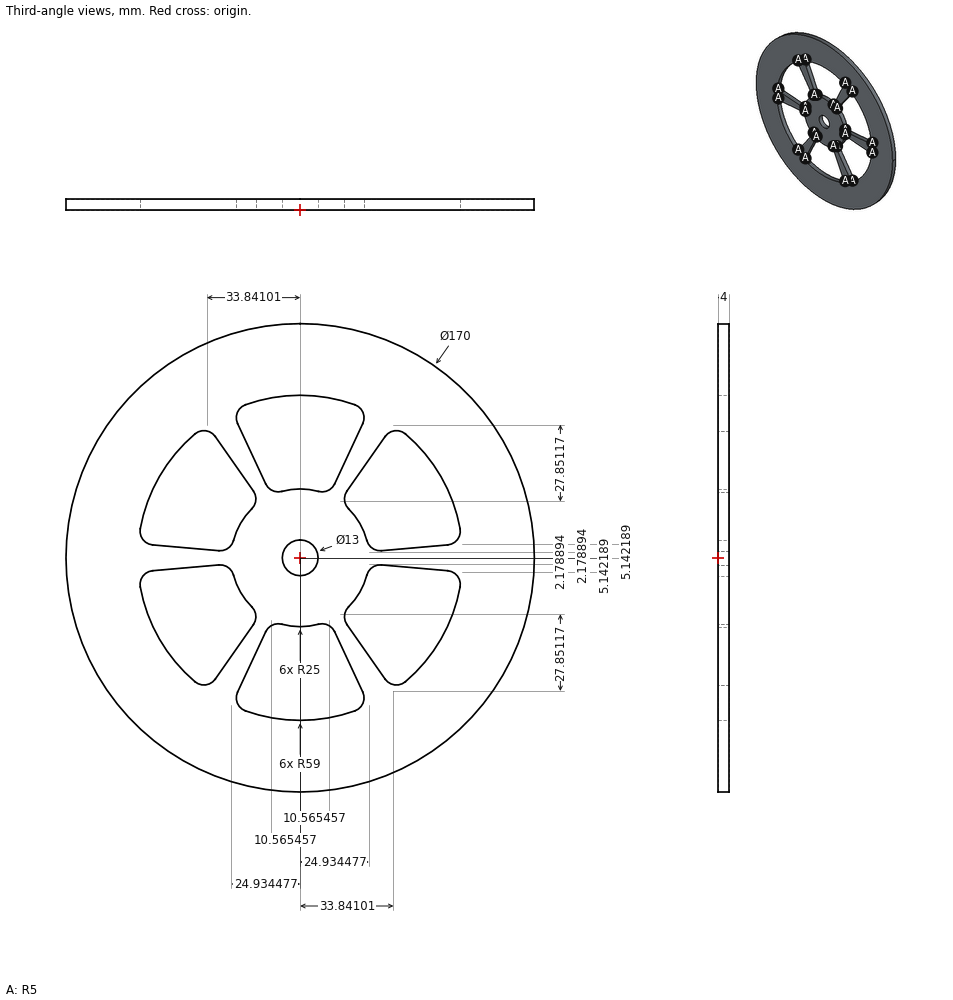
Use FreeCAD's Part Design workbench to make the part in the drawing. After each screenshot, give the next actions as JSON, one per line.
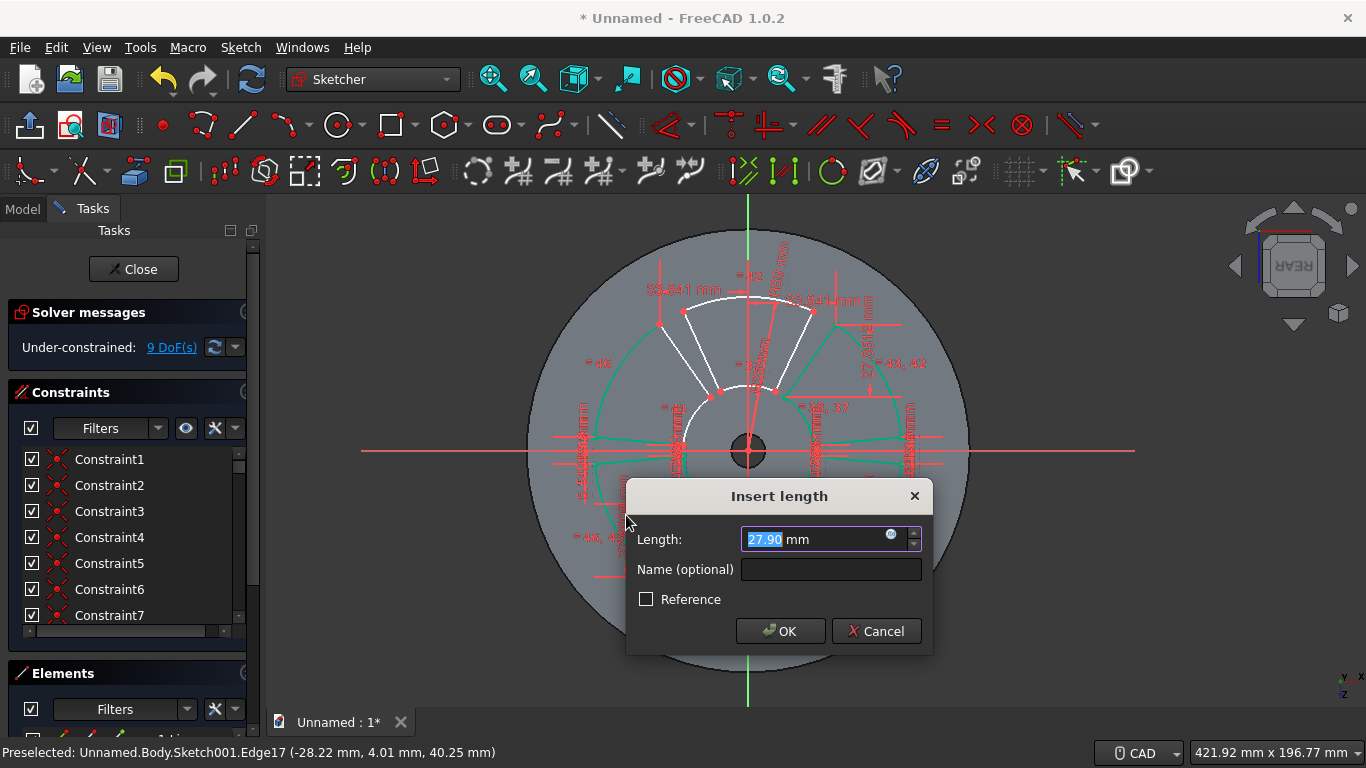
{"action": "type", "text": "27.85117"}
{"action": "key", "text": "Return"}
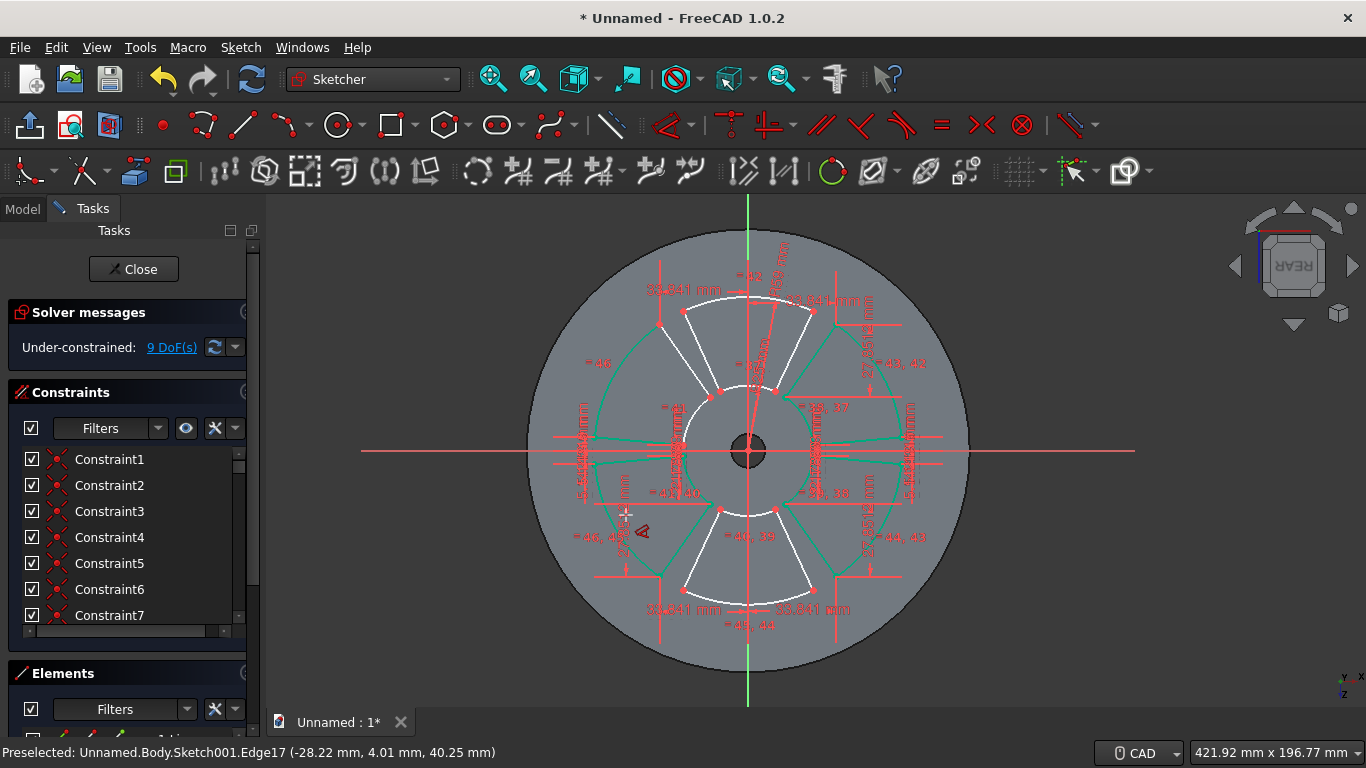
{"action": "left_click", "coordinate": [695, 376]}
{"action": "left_click", "coordinate": [626, 336]}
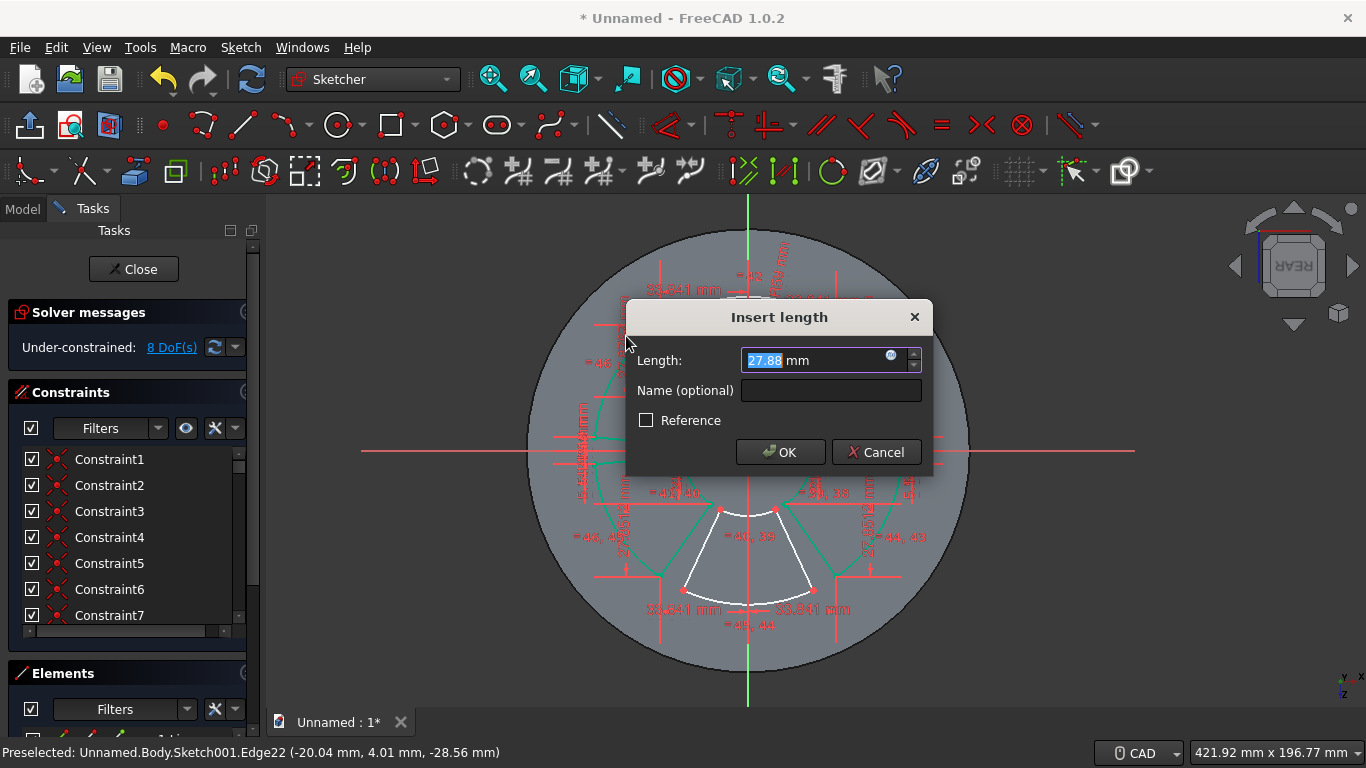
{"action": "type", "text": "27.85117"}
{"action": "key", "text": "Return"}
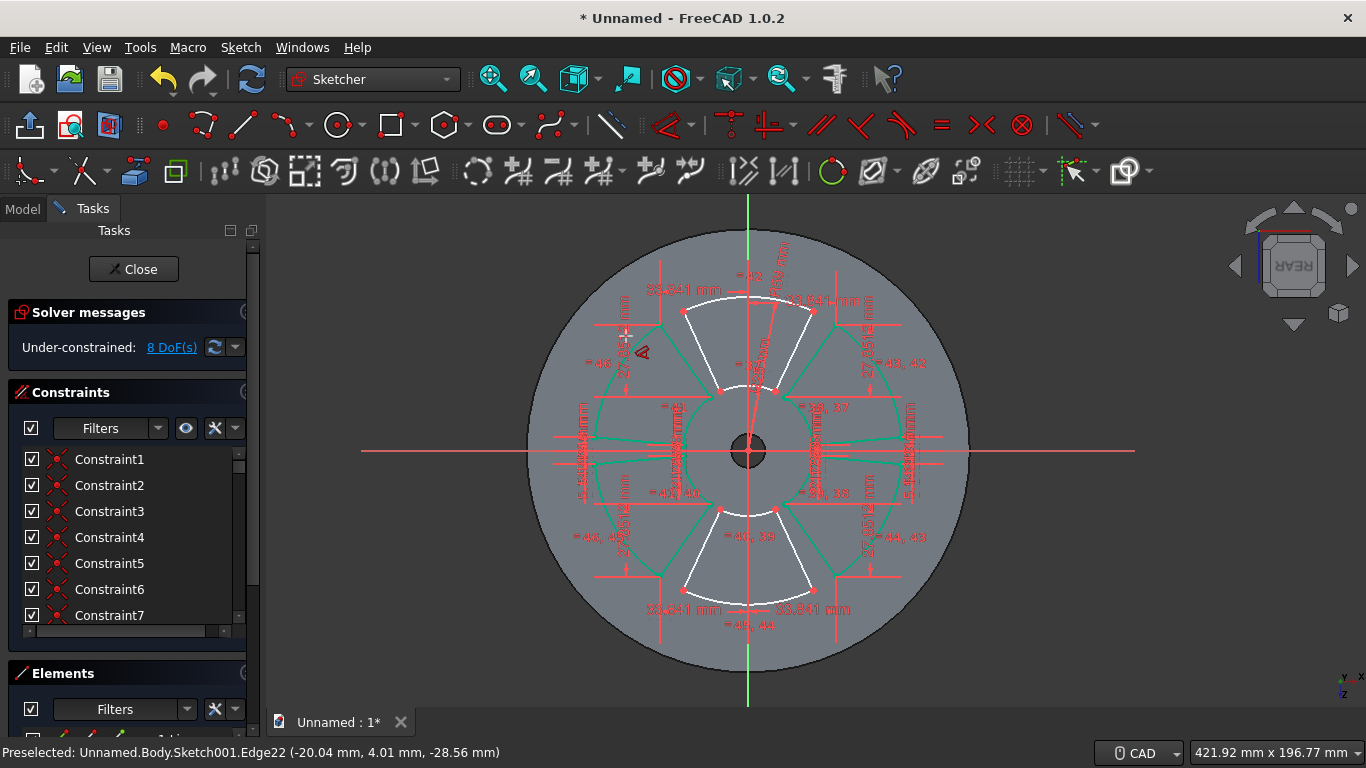
{"action": "scroll", "coordinate": [775, 392], "scroll_direction": "up", "scroll_amount": 2}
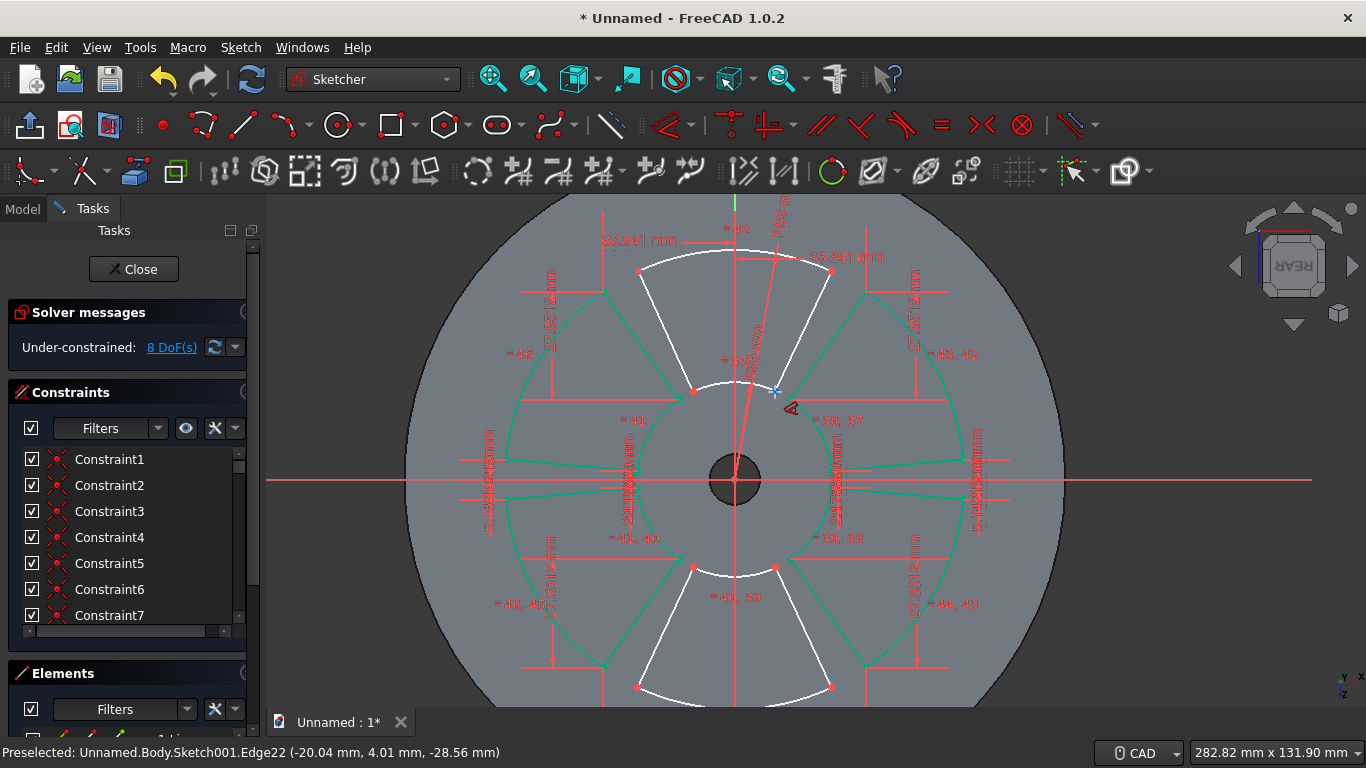
{"action": "left_click", "coordinate": [775, 391]}
{"action": "left_click", "coordinate": [755, 514]}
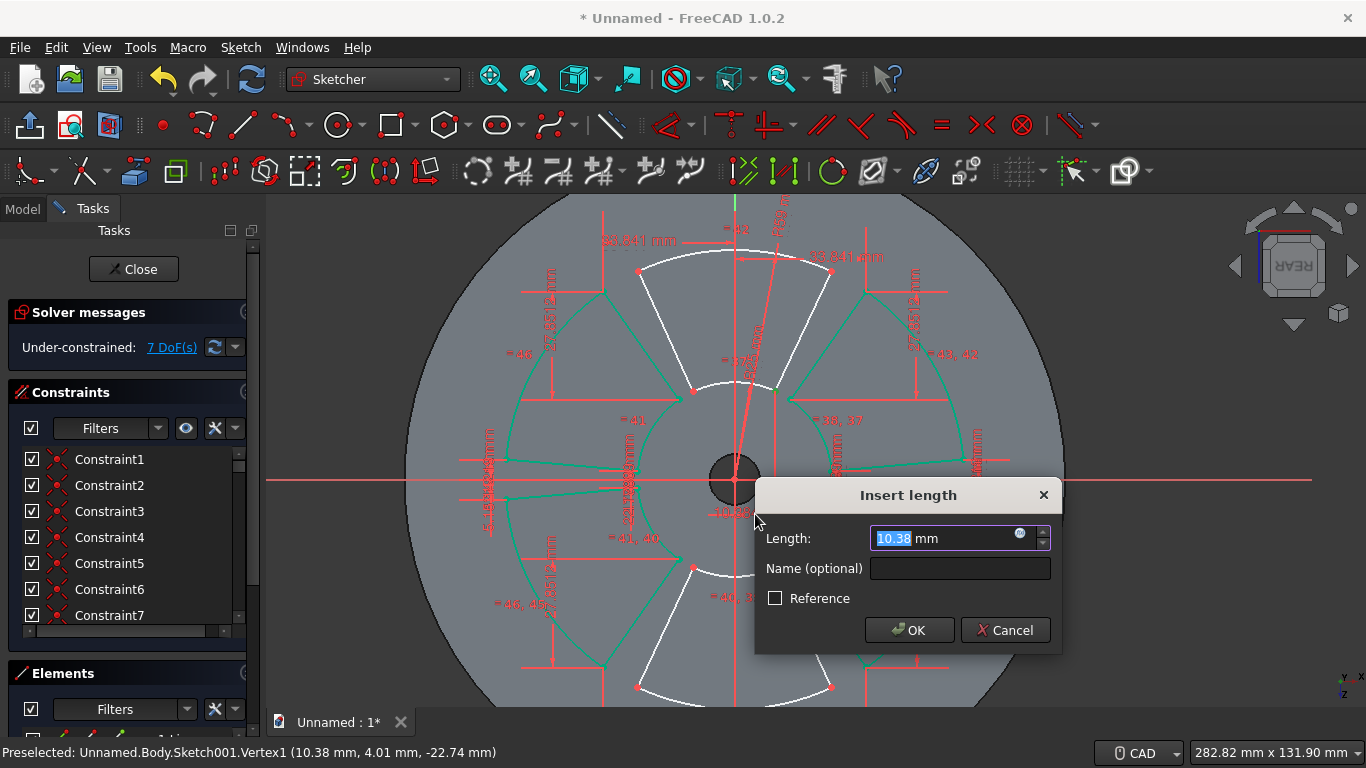
{"action": "type", "text": "10.565457"}
{"action": "key", "text": "Return"}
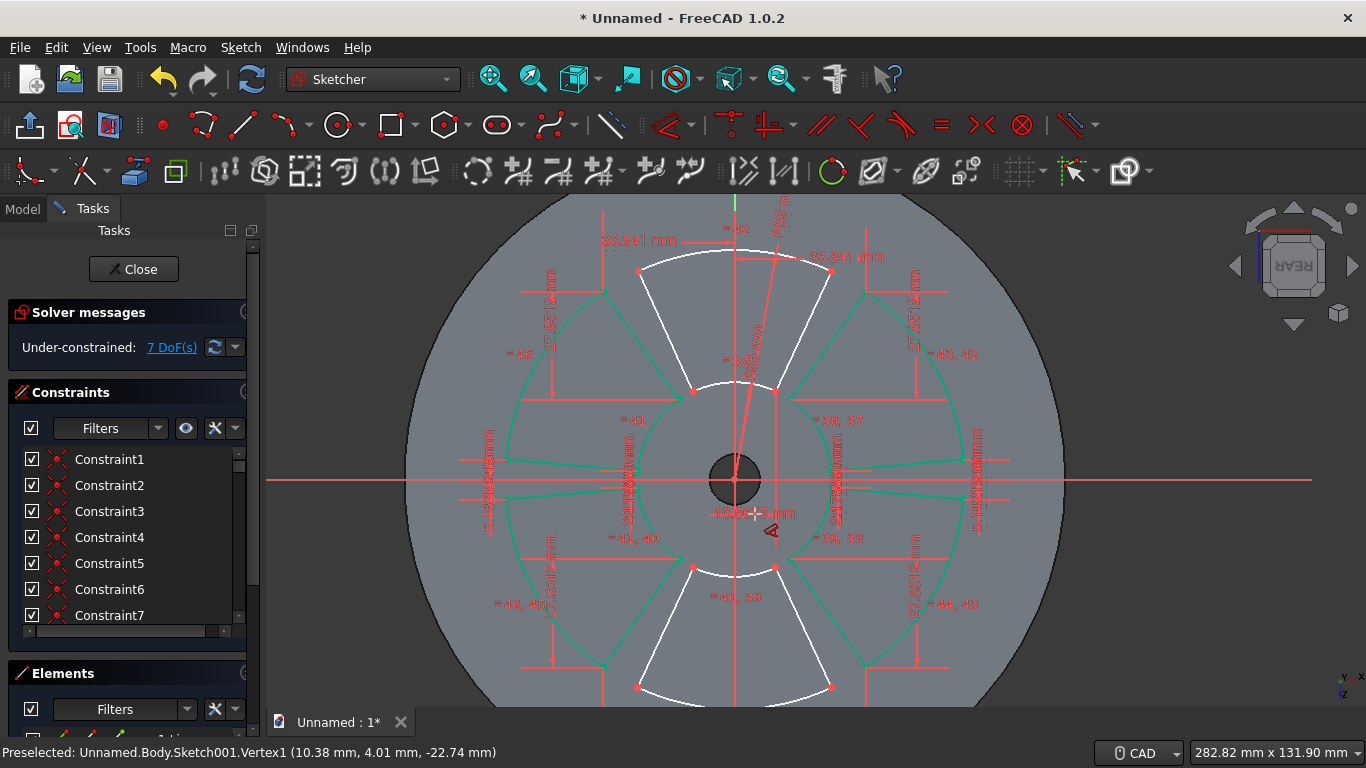
{"action": "left_click", "coordinate": [832, 271]}
{"action": "left_click", "coordinate": [783, 237]}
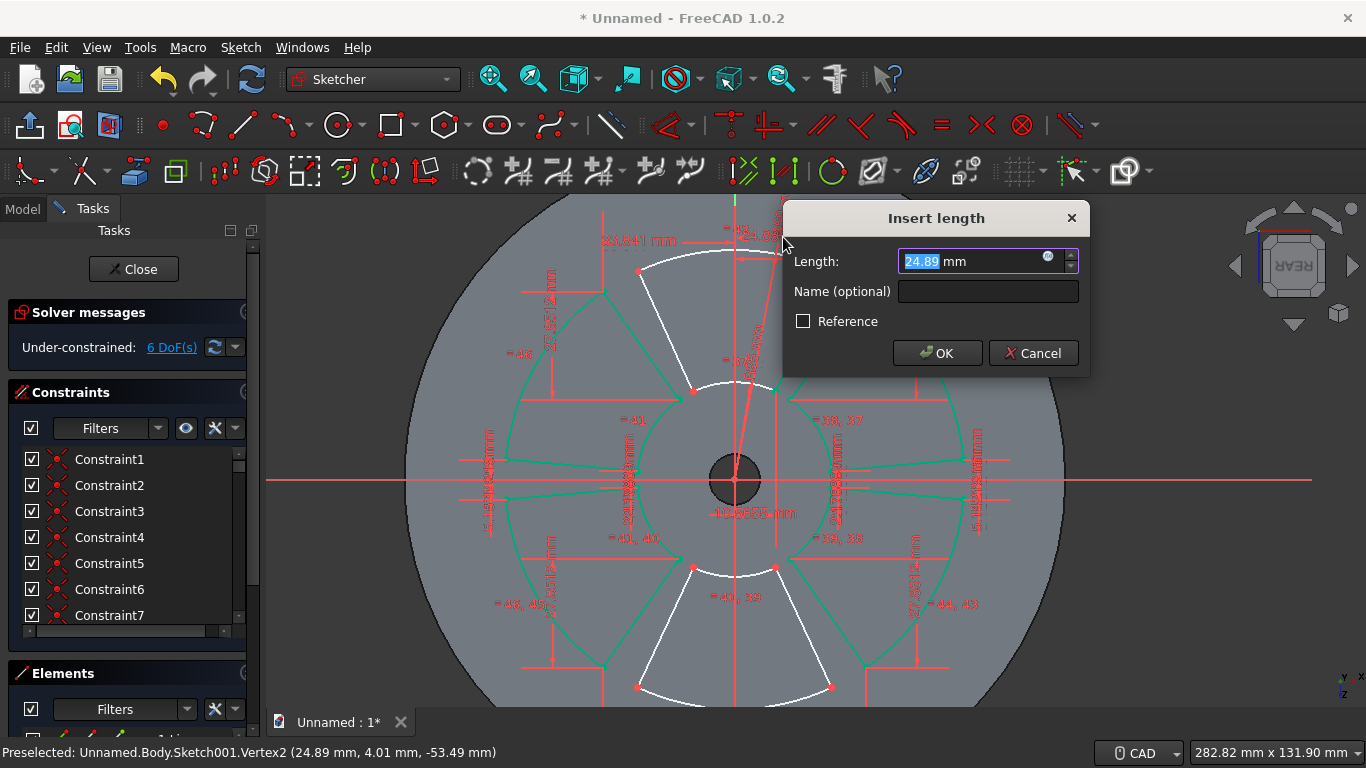
{"action": "type", "text": "24.934477"}
{"action": "key", "text": "Return"}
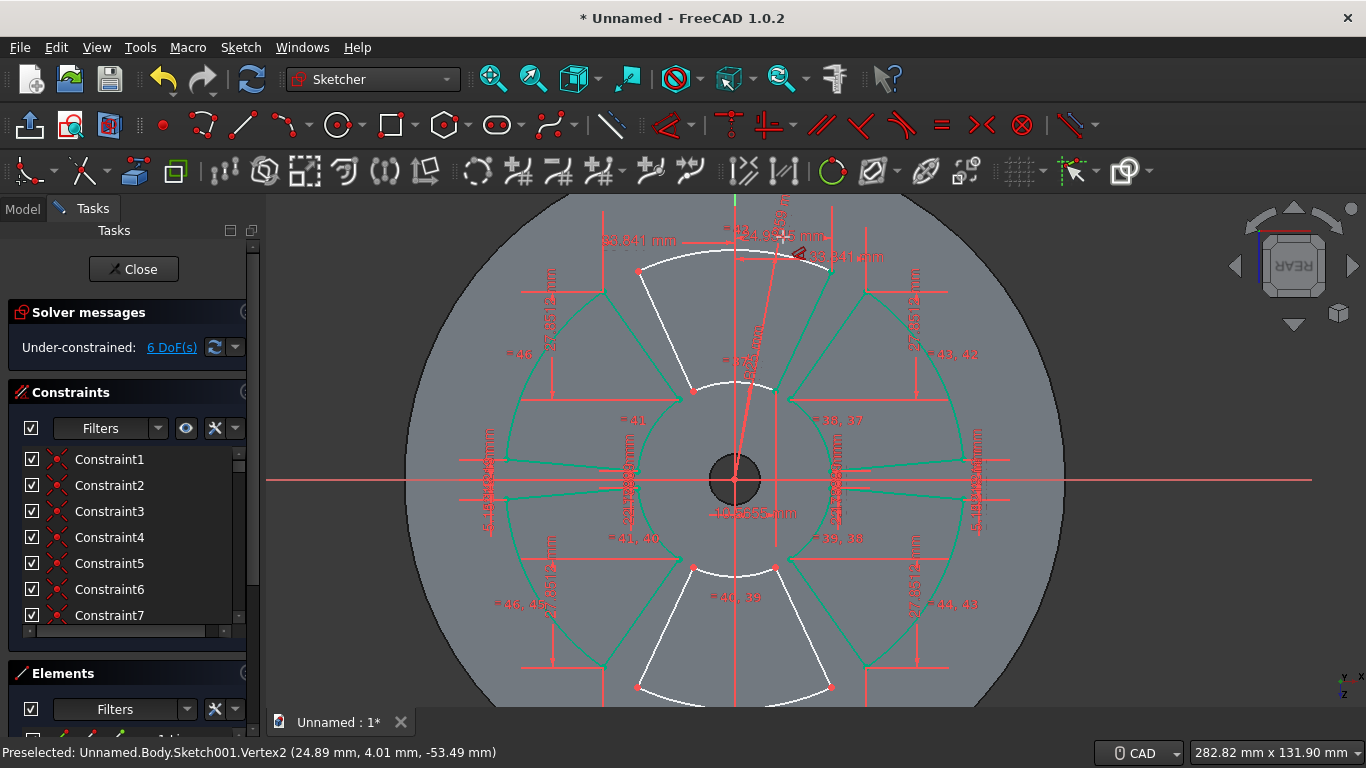
{"action": "left_click", "coordinate": [638, 271]}
{"action": "left_click", "coordinate": [709, 237]}